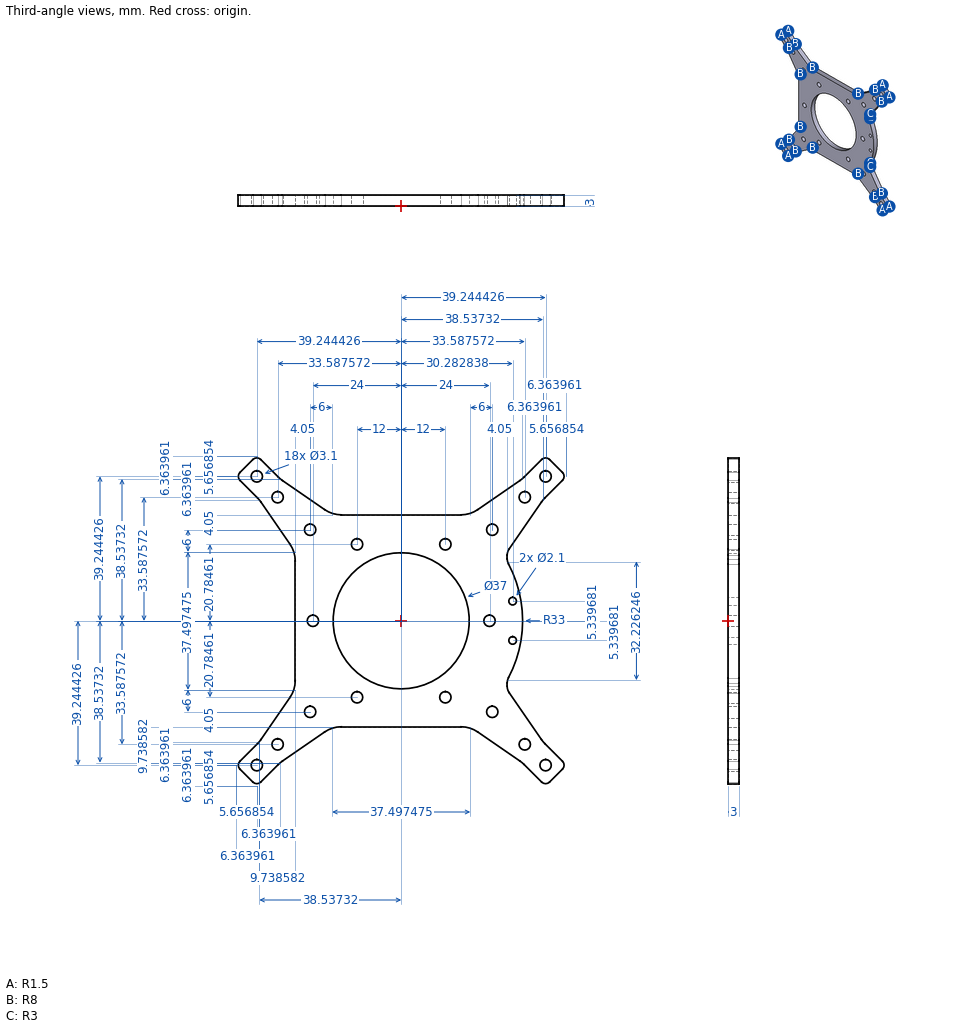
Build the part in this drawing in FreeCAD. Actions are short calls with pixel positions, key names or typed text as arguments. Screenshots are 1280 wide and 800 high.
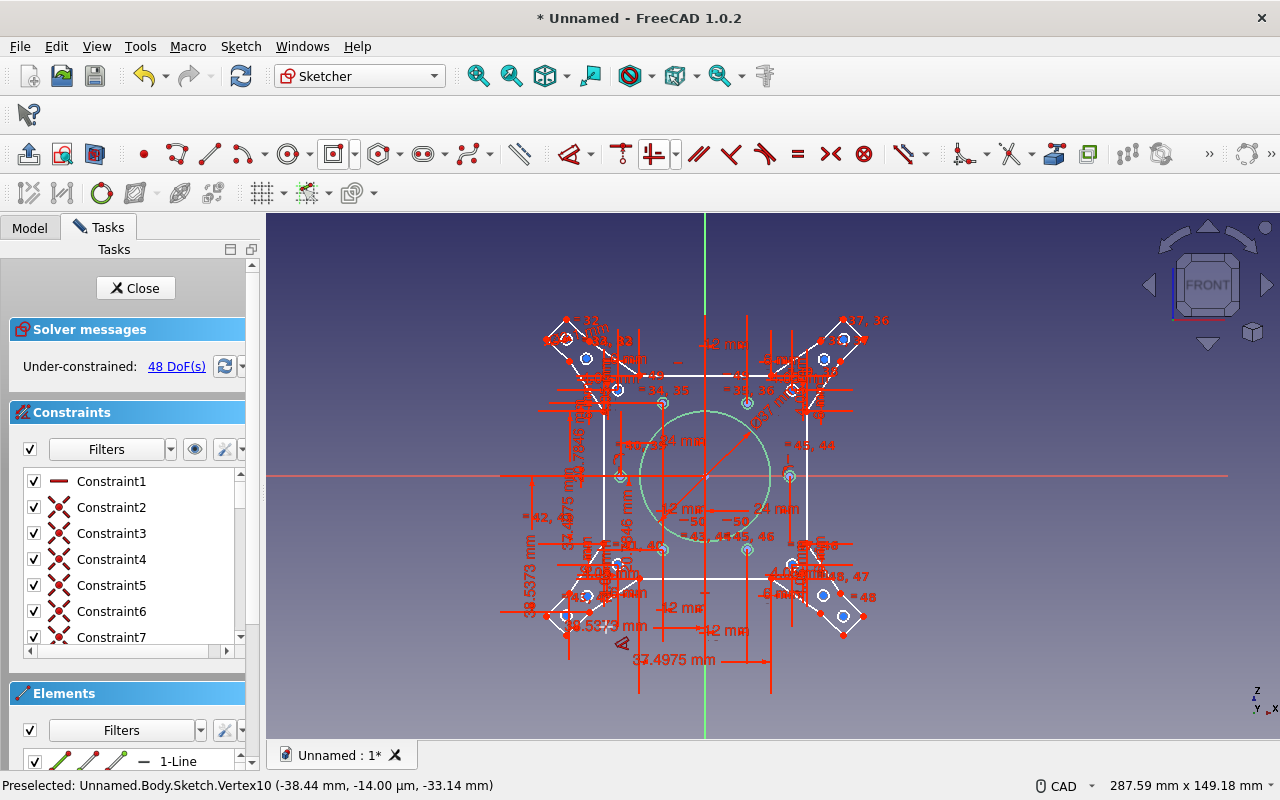
click(570, 361)
click(637, 303)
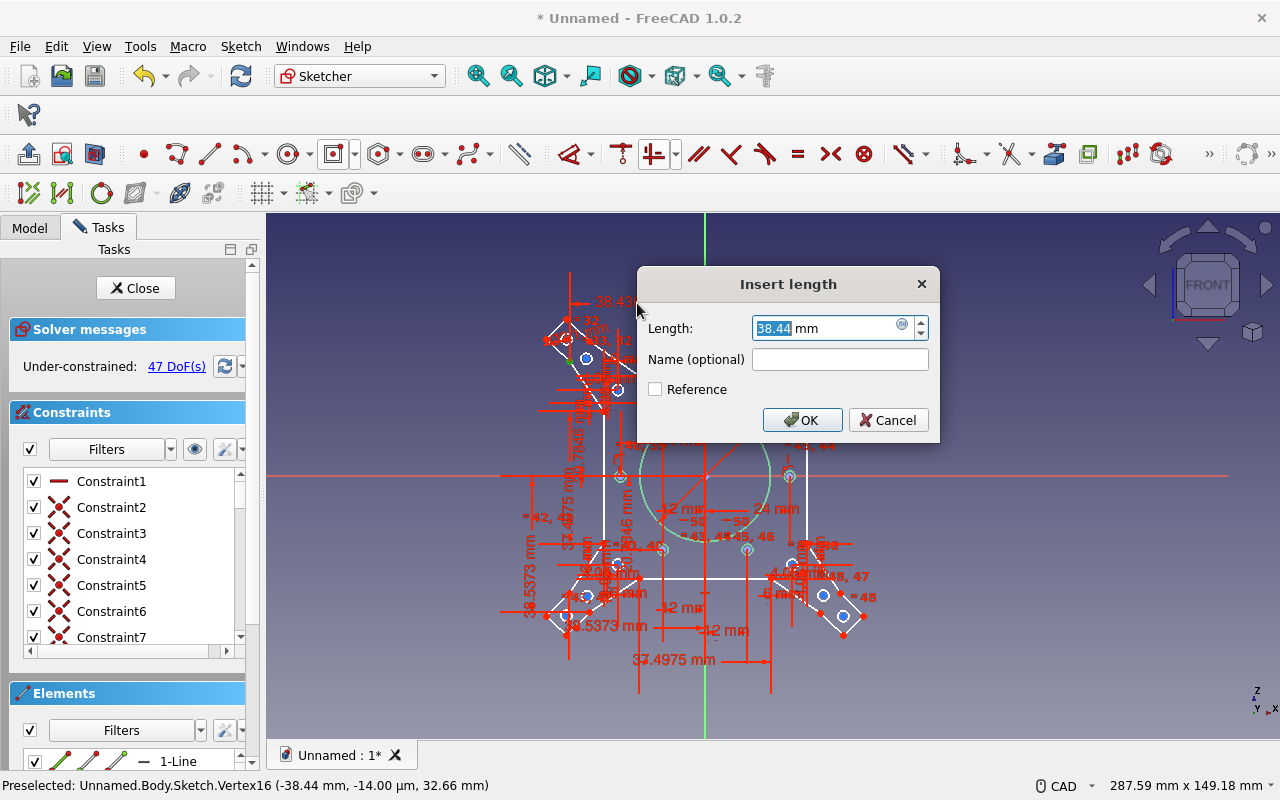
text(38.53732)
key(Return)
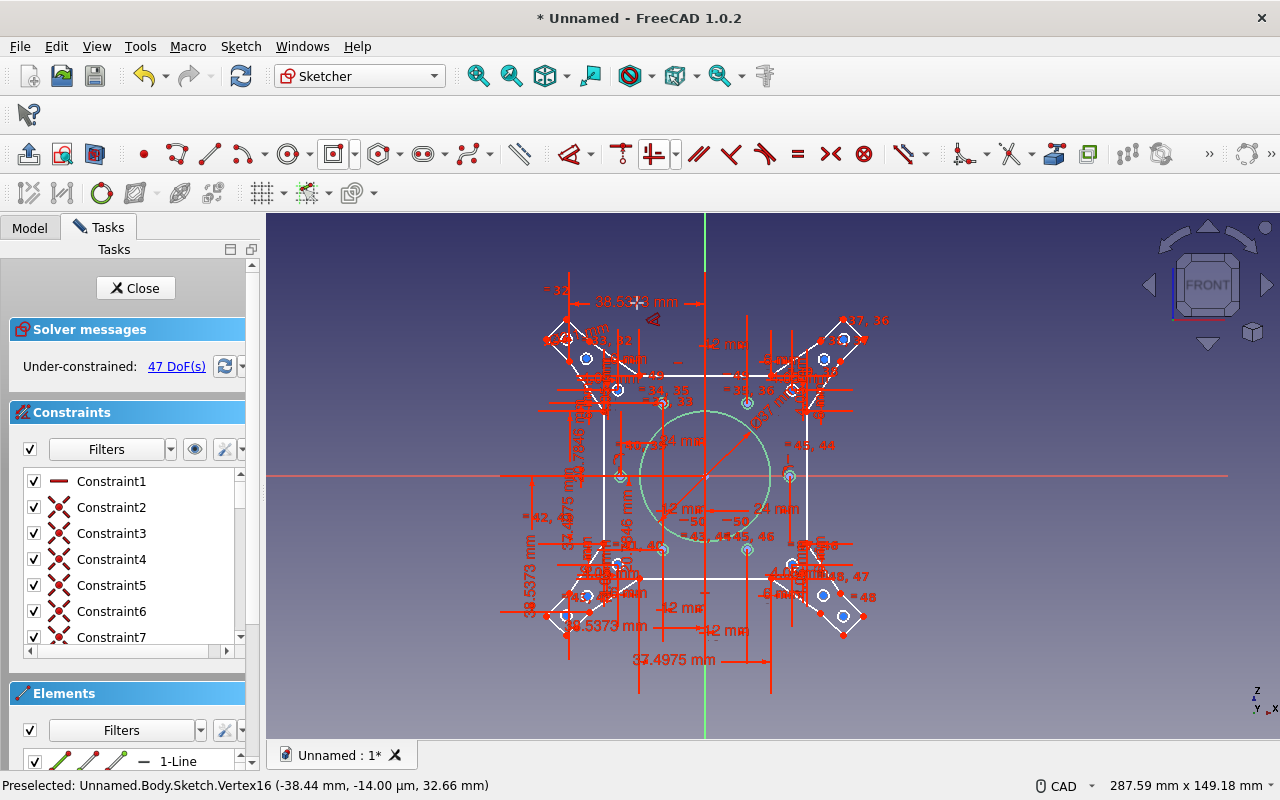
click(590, 341)
click(532, 378)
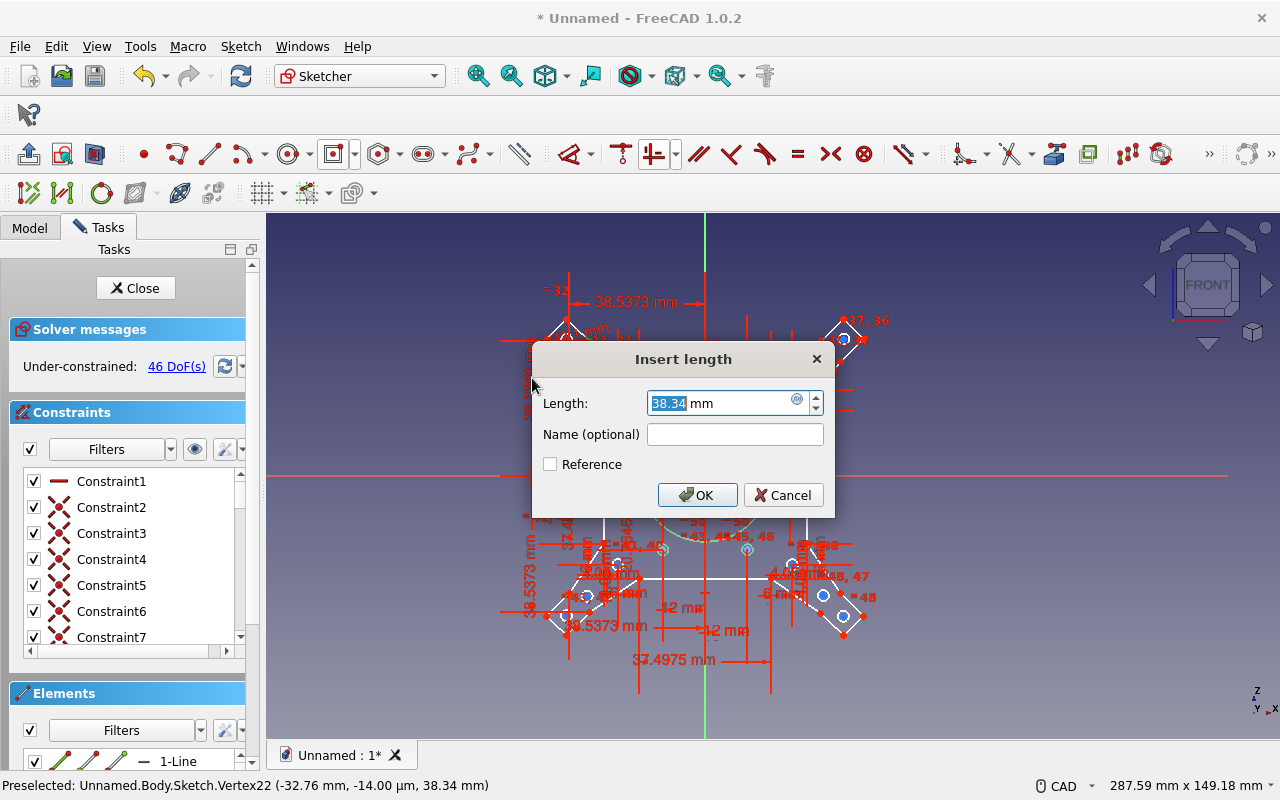
text(38.53732)
key(Return)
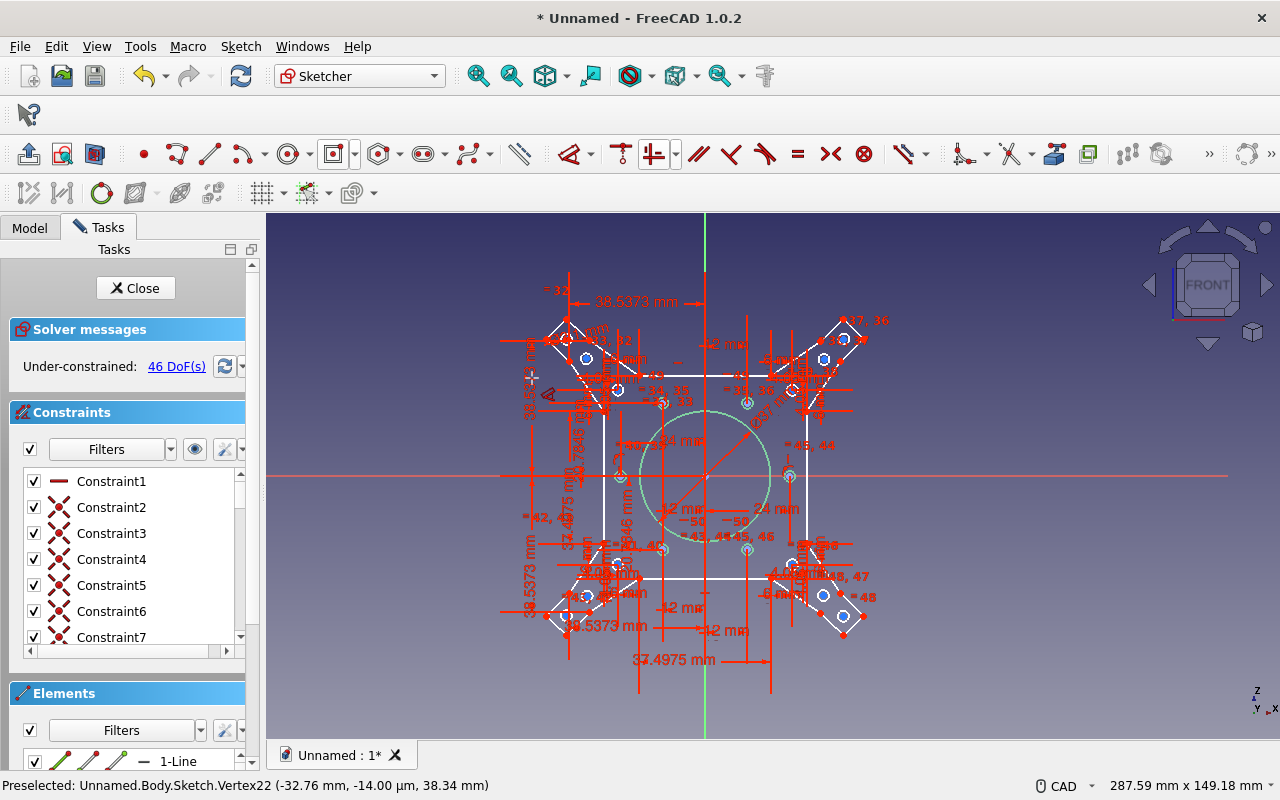
click(821, 341)
click(855, 440)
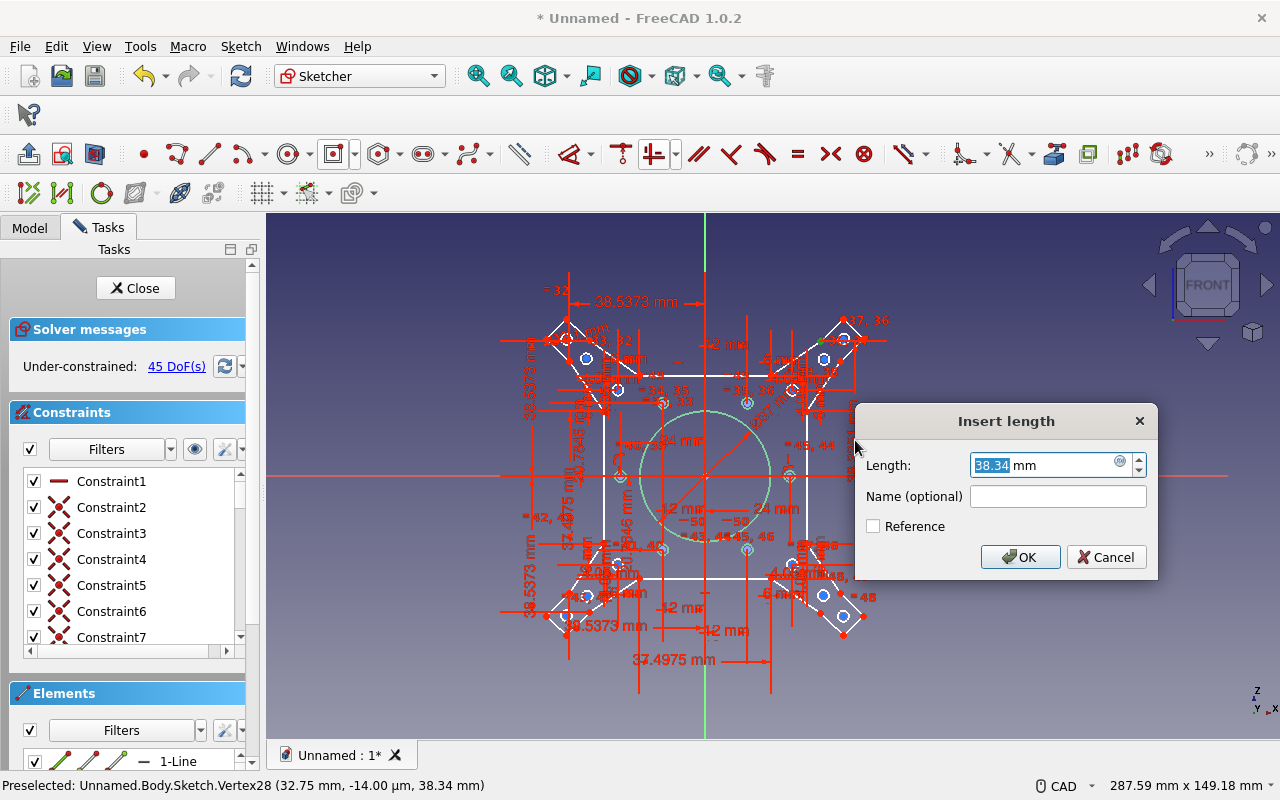
text(38.53732)
key(Return)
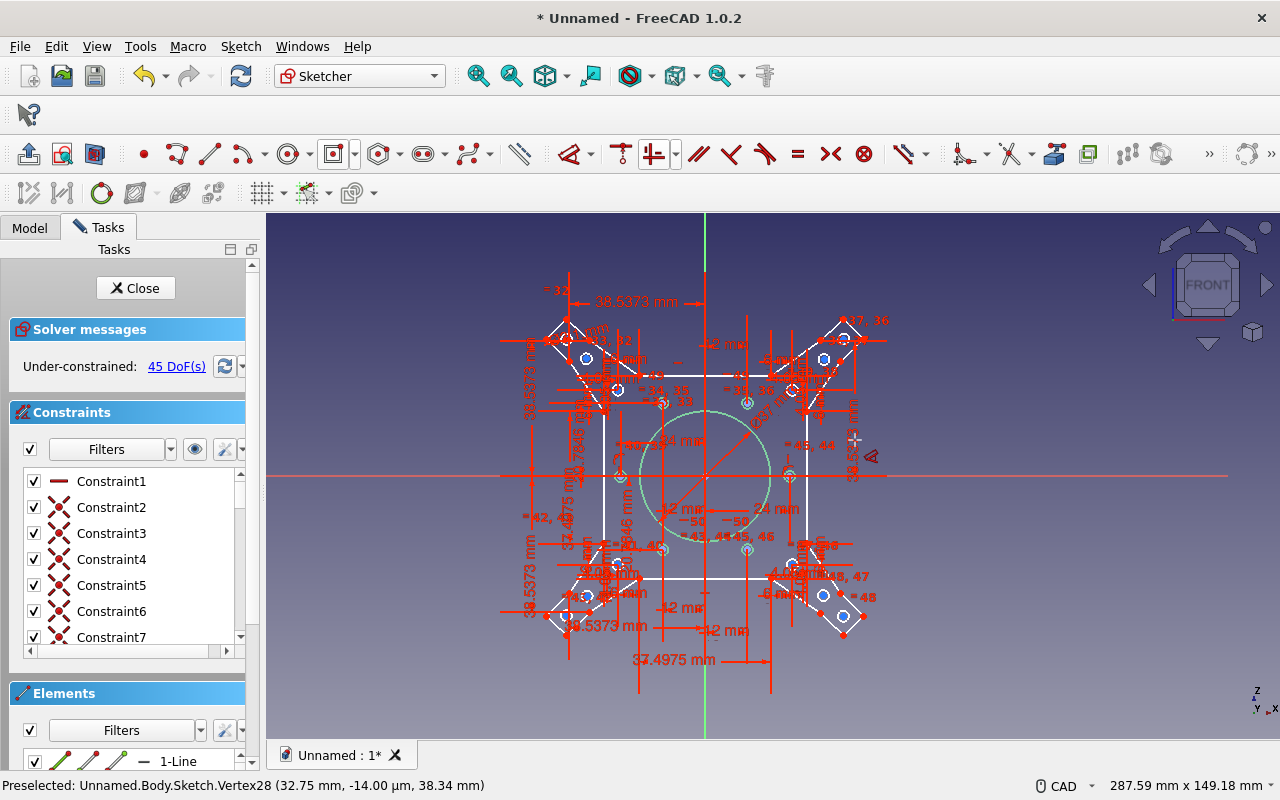
click(841, 361)
click(804, 327)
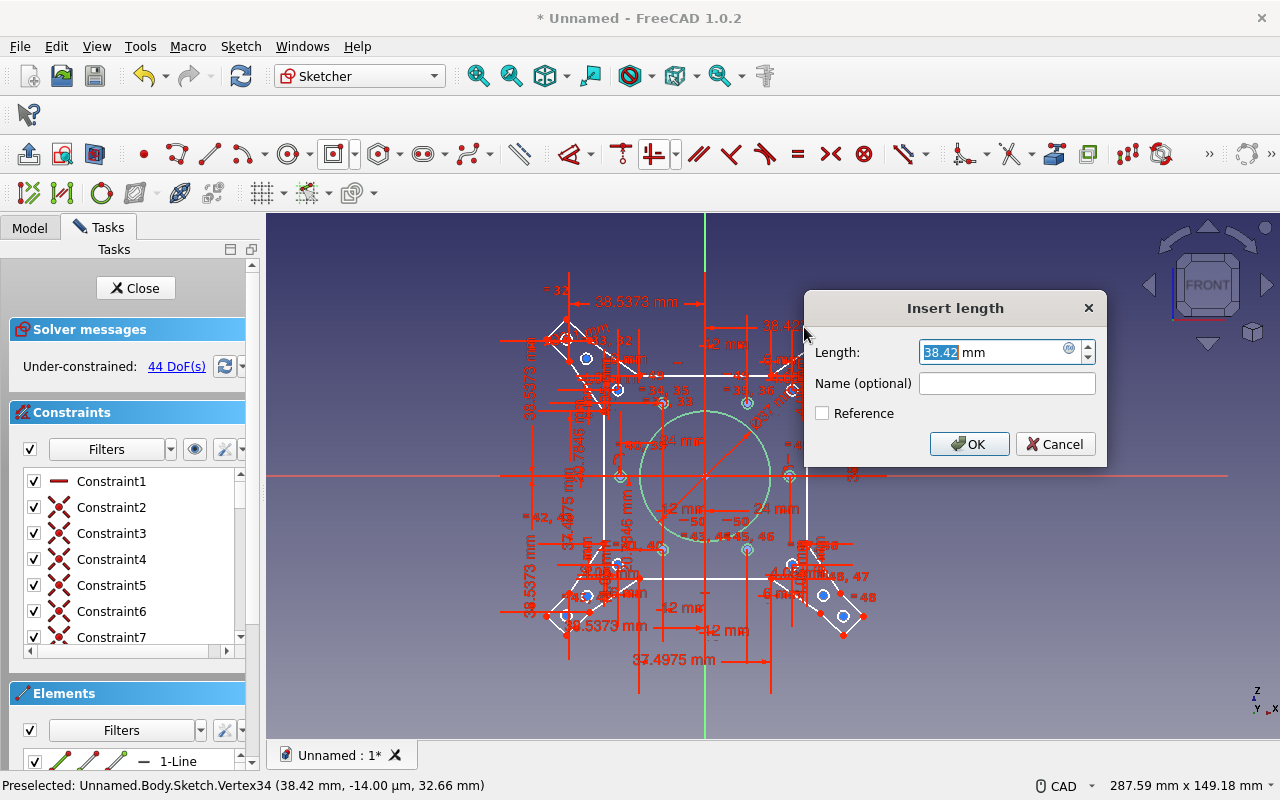
text(38.53732)
key(Return)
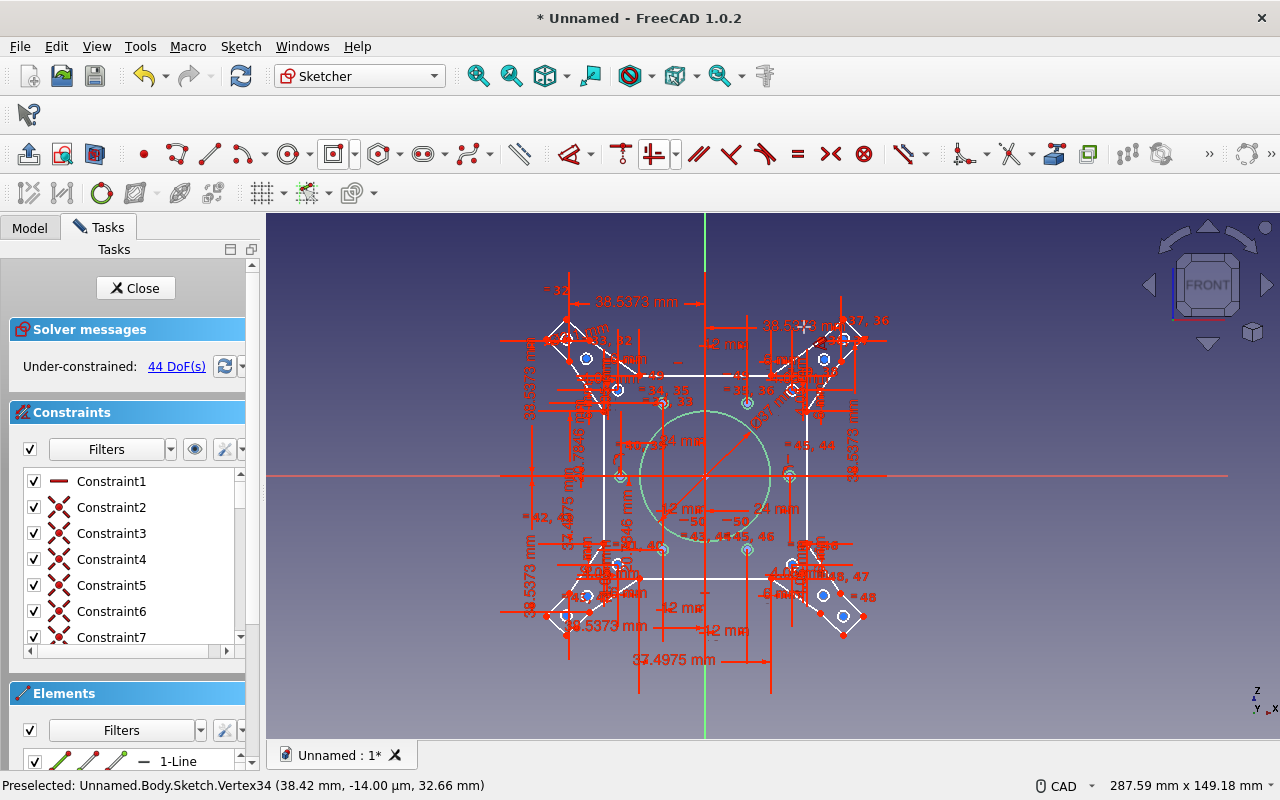
click(841, 593)
click(804, 627)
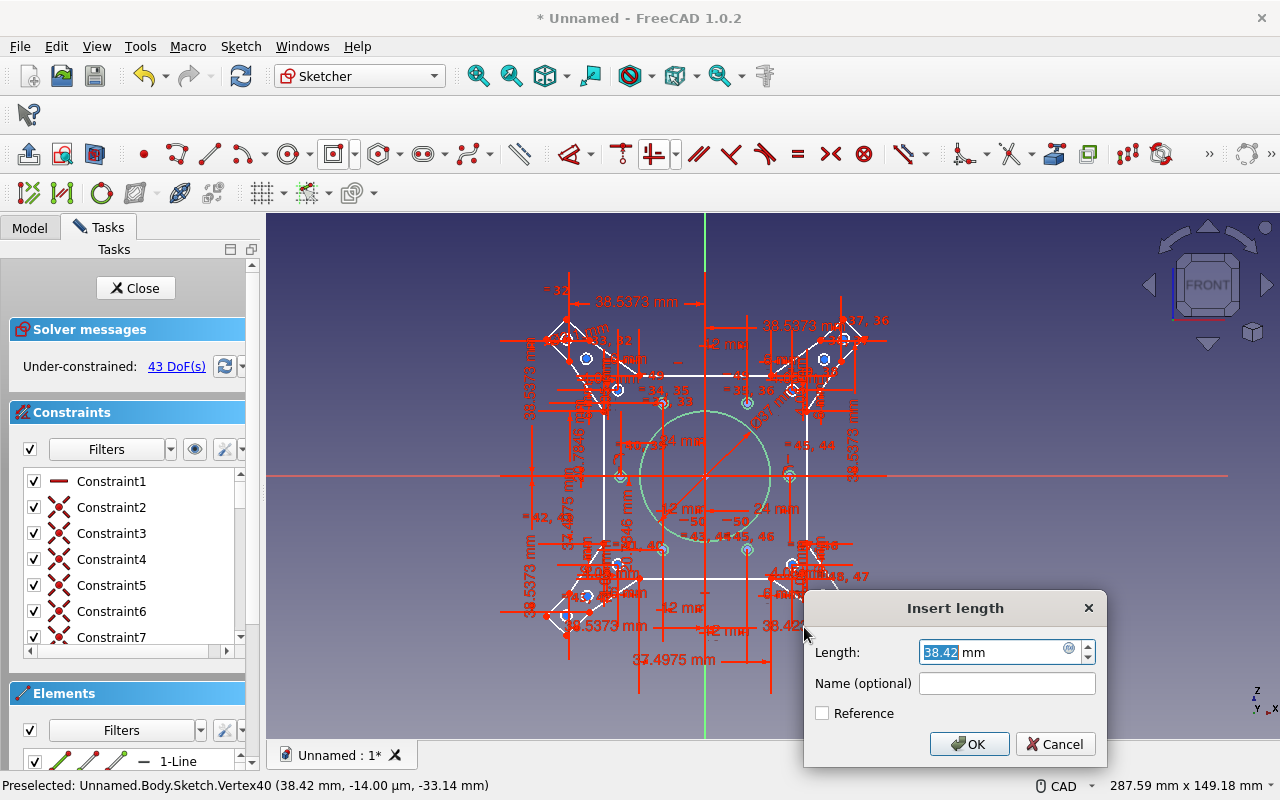
text(38.53732)
key(Return)